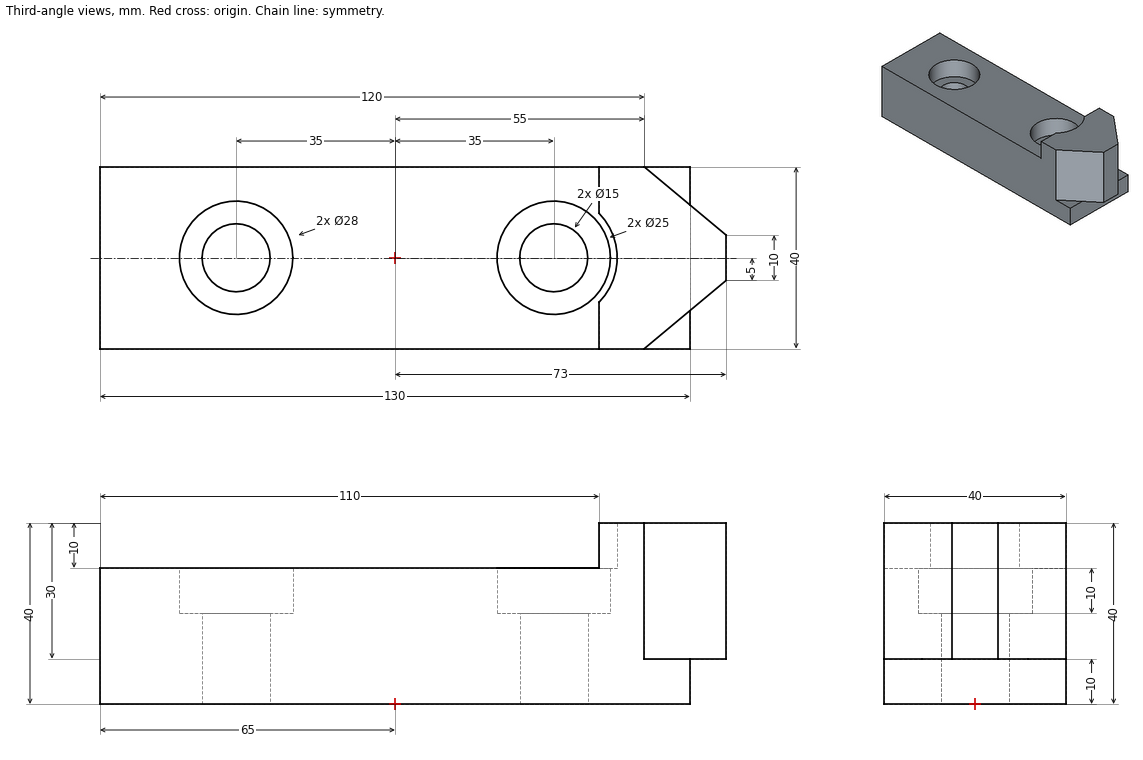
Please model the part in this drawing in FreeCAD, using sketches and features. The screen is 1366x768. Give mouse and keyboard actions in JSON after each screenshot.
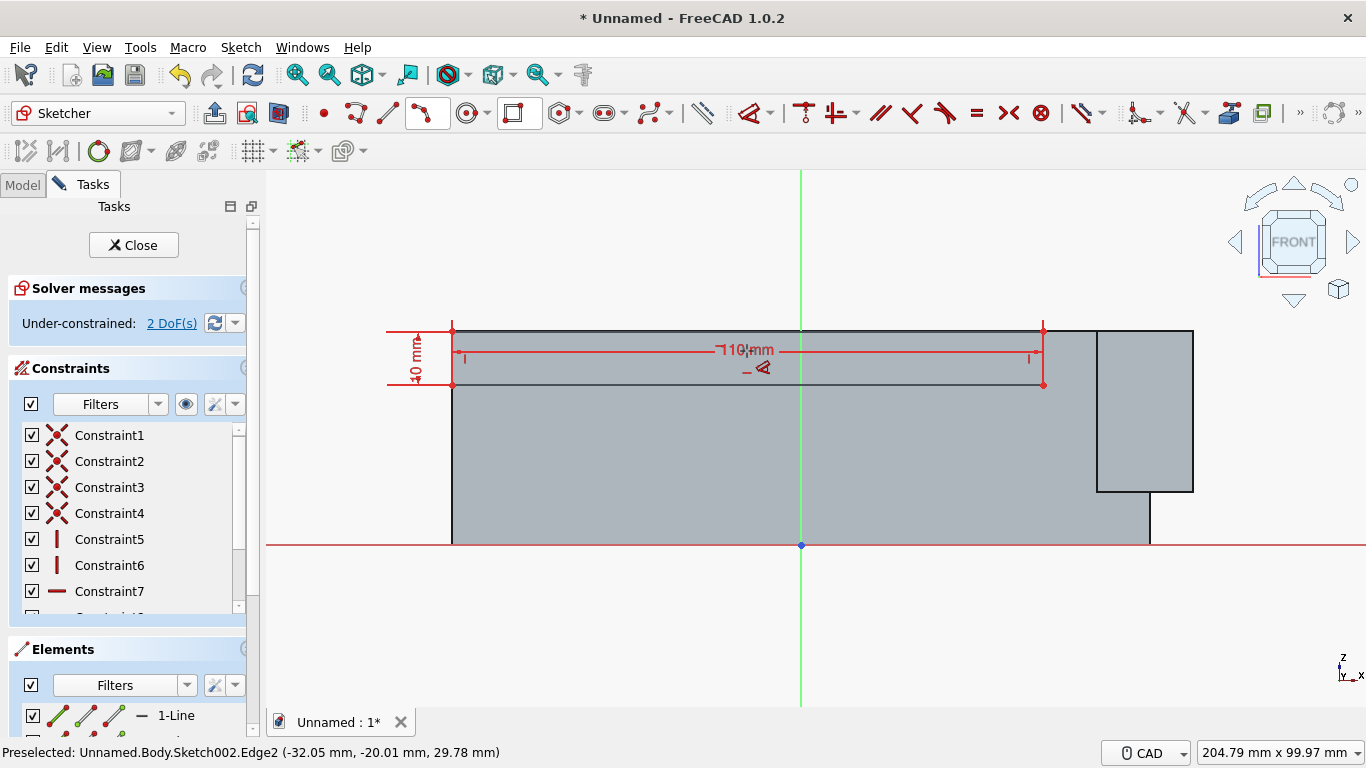
{"action": "left_click", "coordinate": [452, 332]}
{"action": "left_click", "coordinate": [627, 579]}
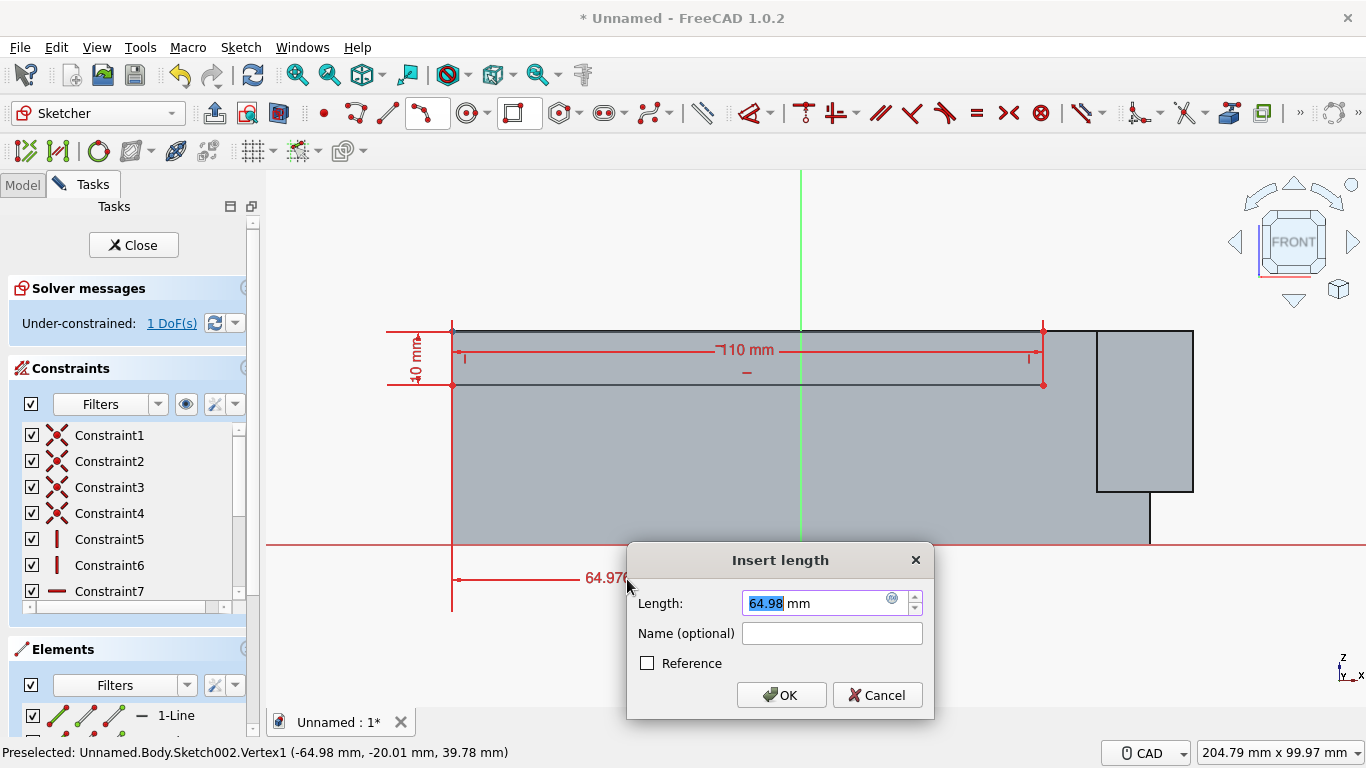
{"action": "type", "text": "65"}
{"action": "key", "text": "Return"}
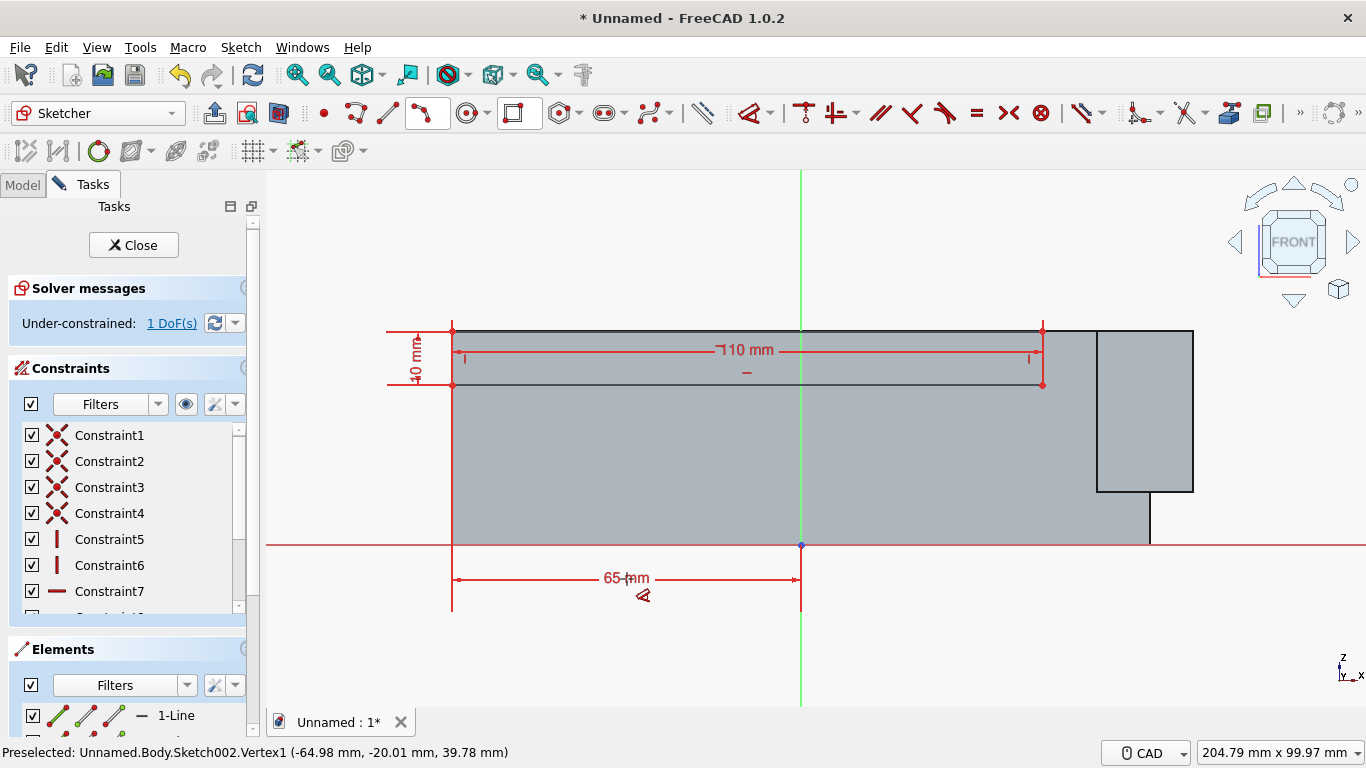
{"action": "left_click", "coordinate": [452, 332]}
{"action": "left_click", "coordinate": [418, 439]}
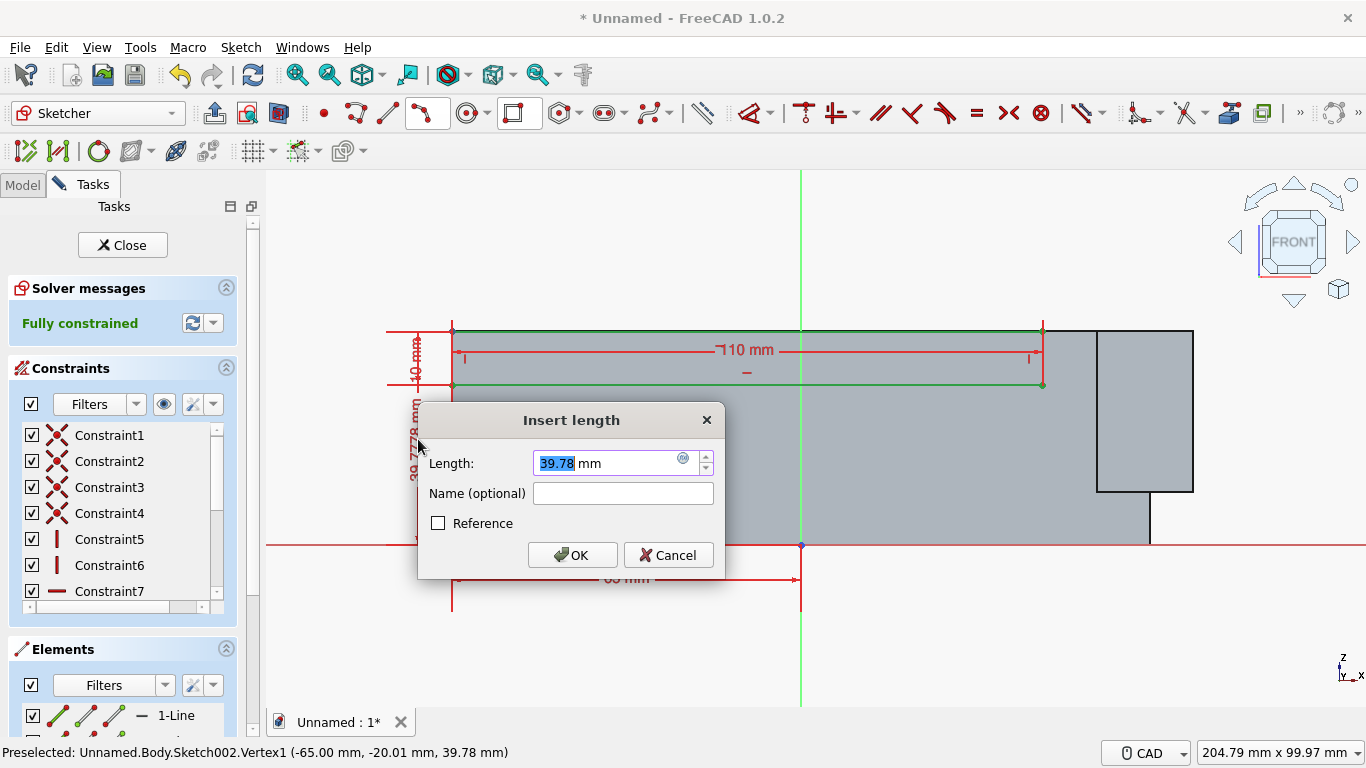
{"action": "type", "text": "40"}
{"action": "key", "text": "Return"}
{"action": "key", "text": "Escape"}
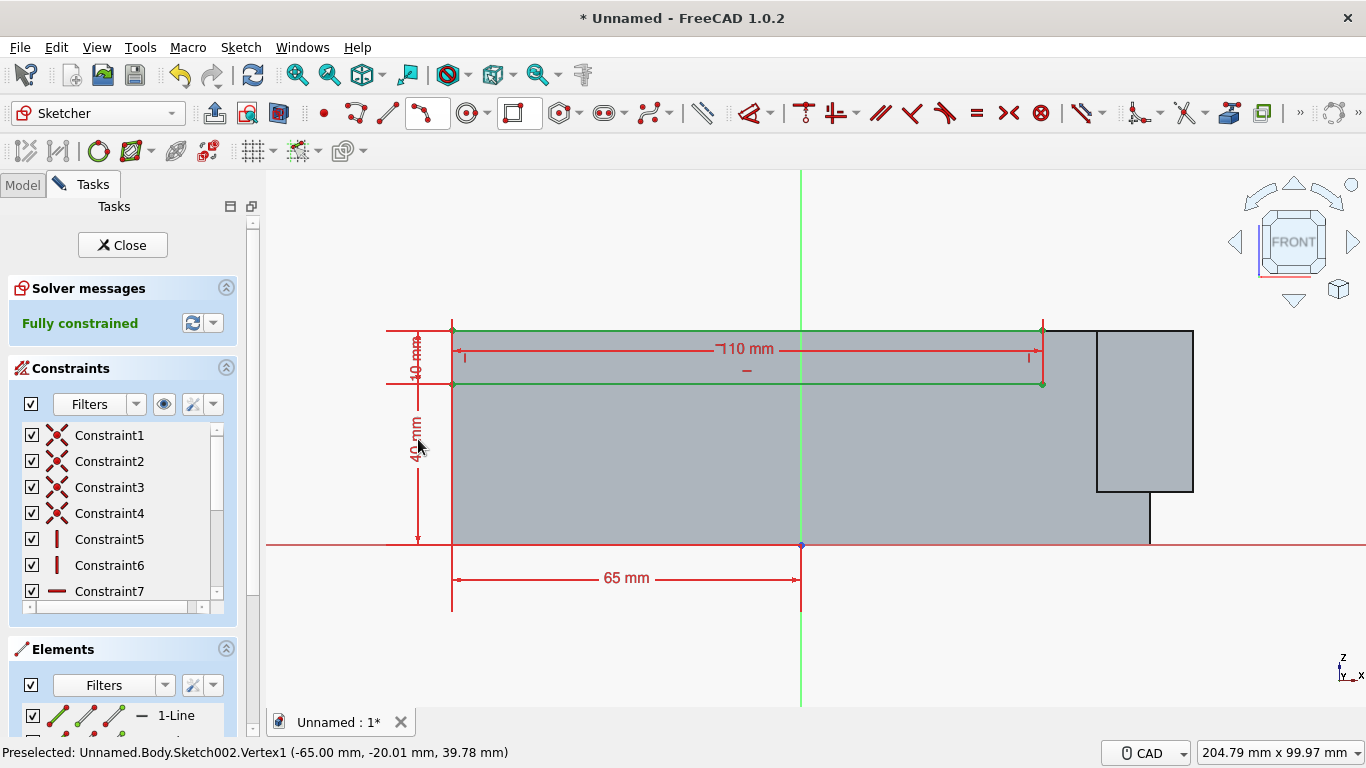
{"action": "left_click", "coordinate": [123, 245]}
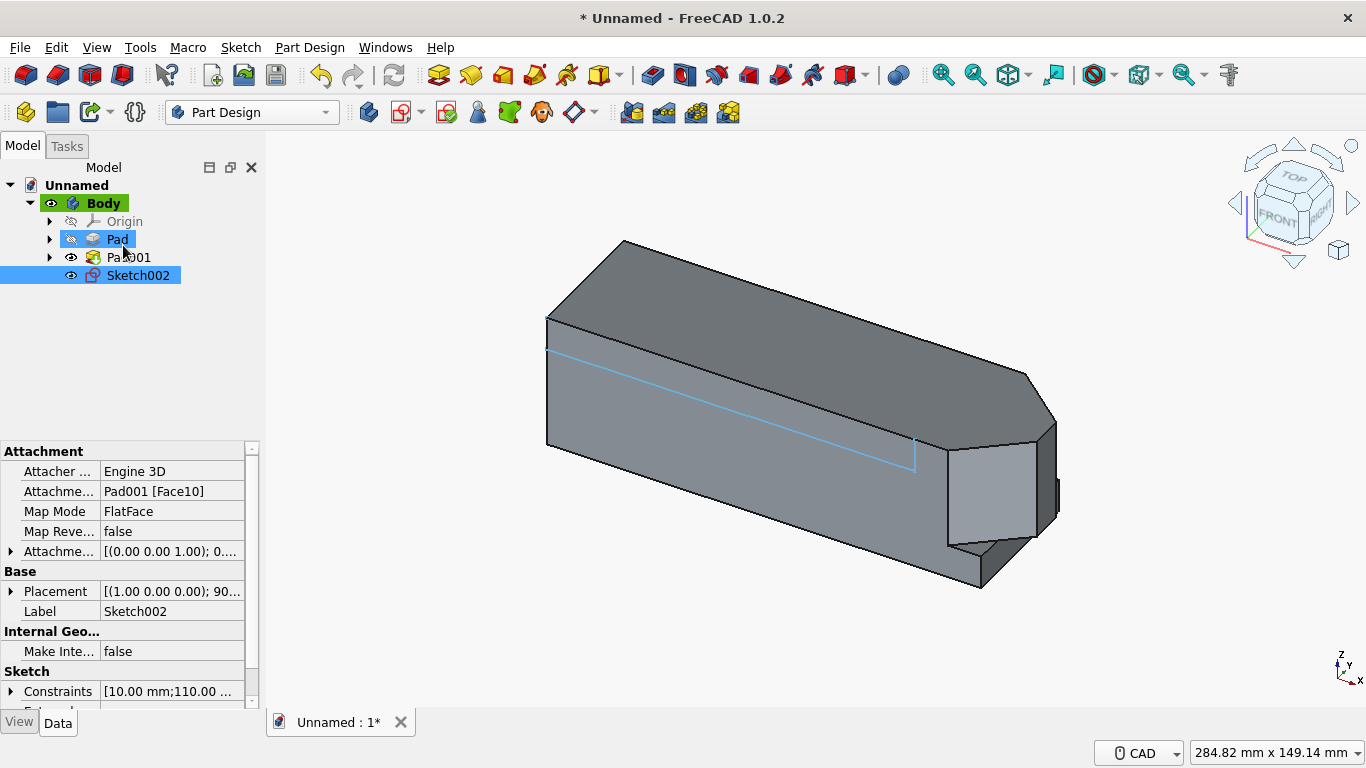
{"action": "left_click", "coordinate": [654, 76]}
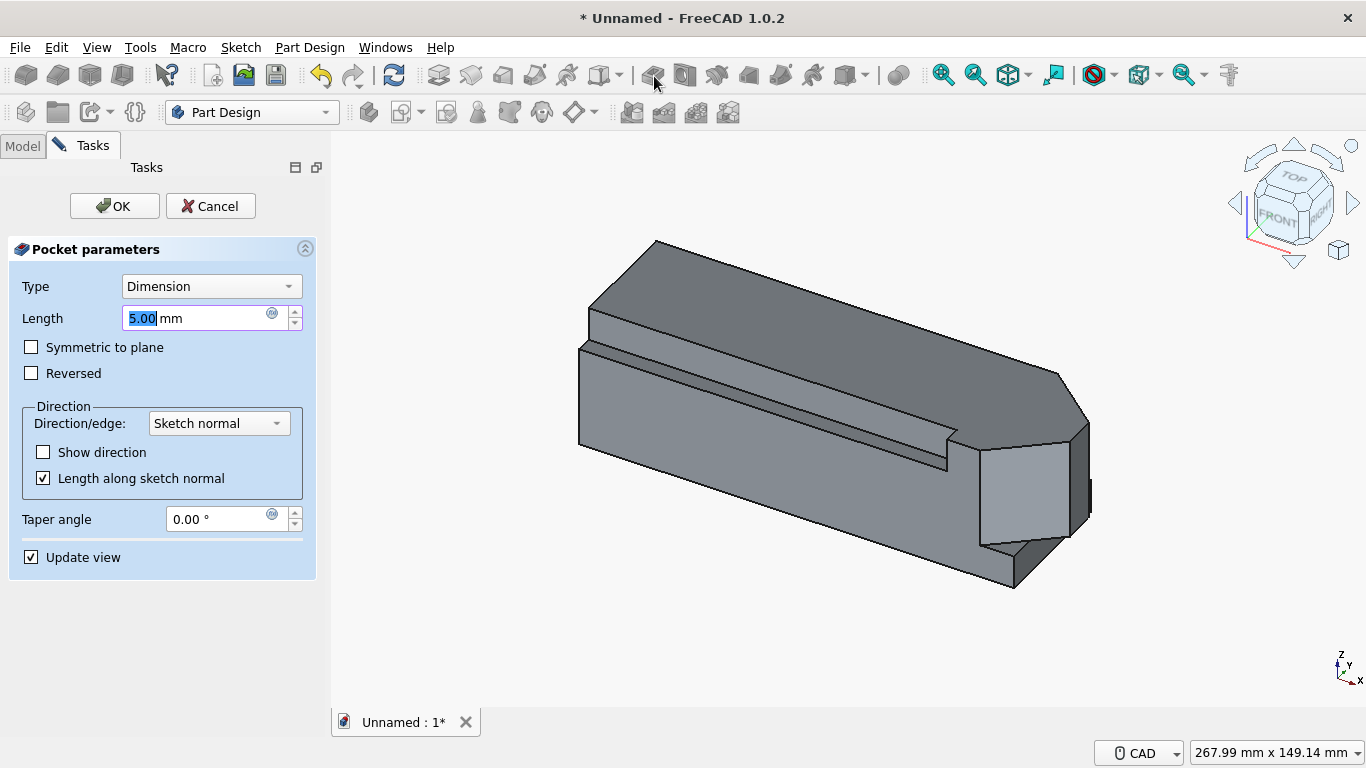
{"action": "type", "text": "40"}
{"action": "key", "text": "Tab"}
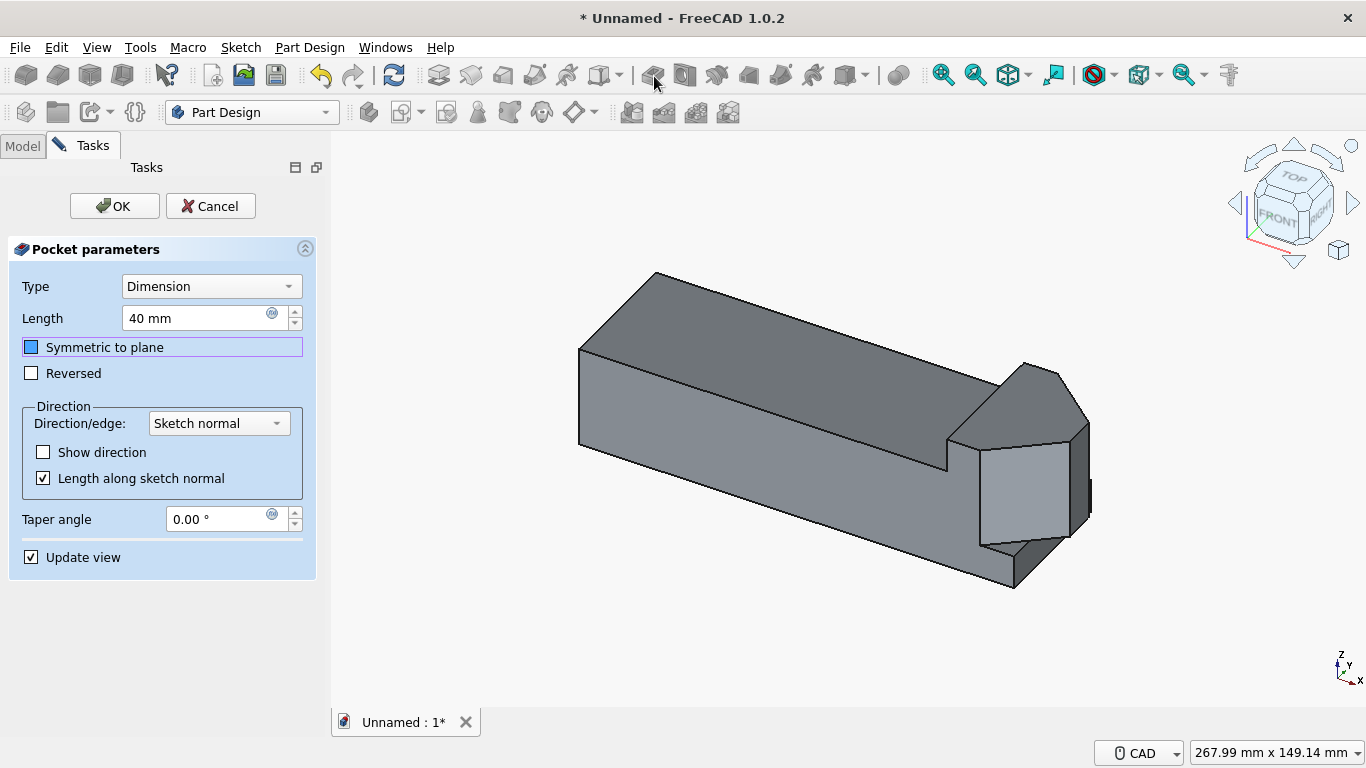
{"action": "left_click", "coordinate": [115, 206]}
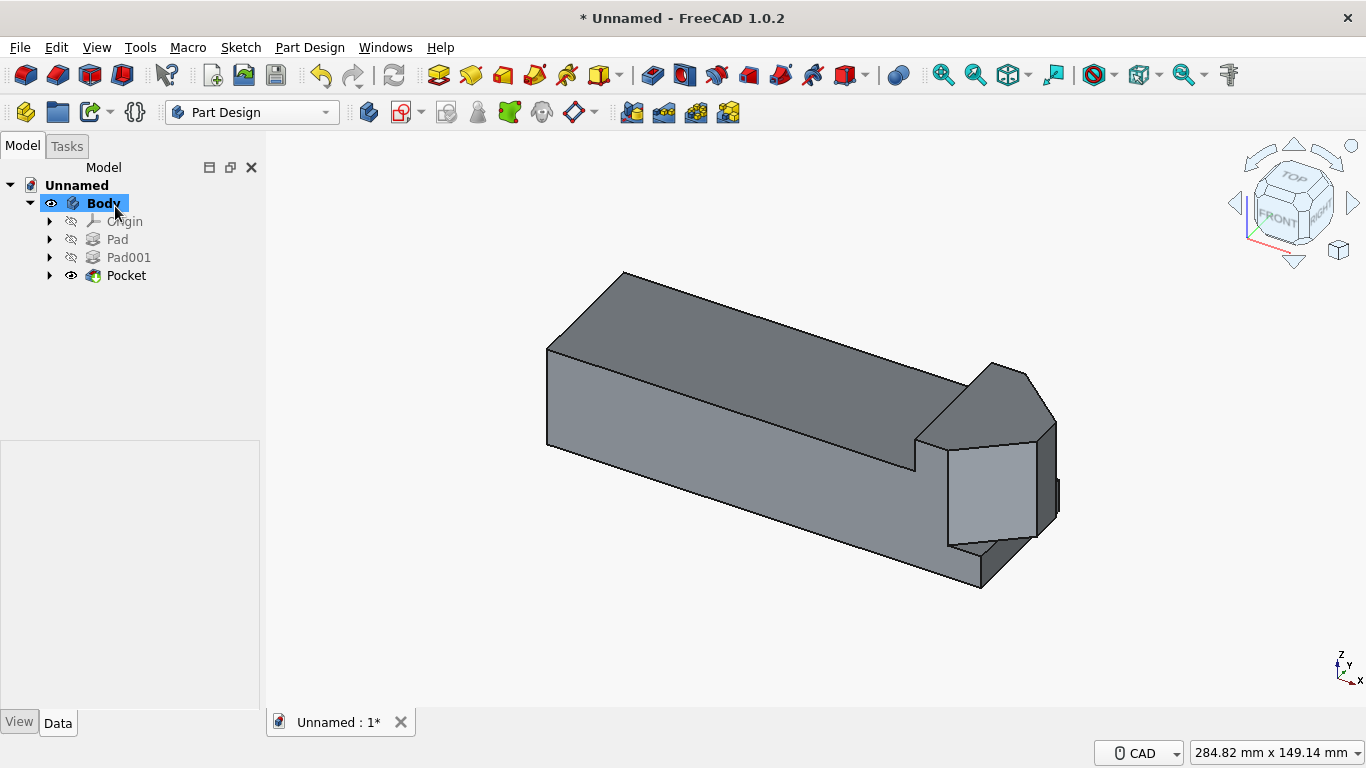
{"action": "key", "text": "5"}